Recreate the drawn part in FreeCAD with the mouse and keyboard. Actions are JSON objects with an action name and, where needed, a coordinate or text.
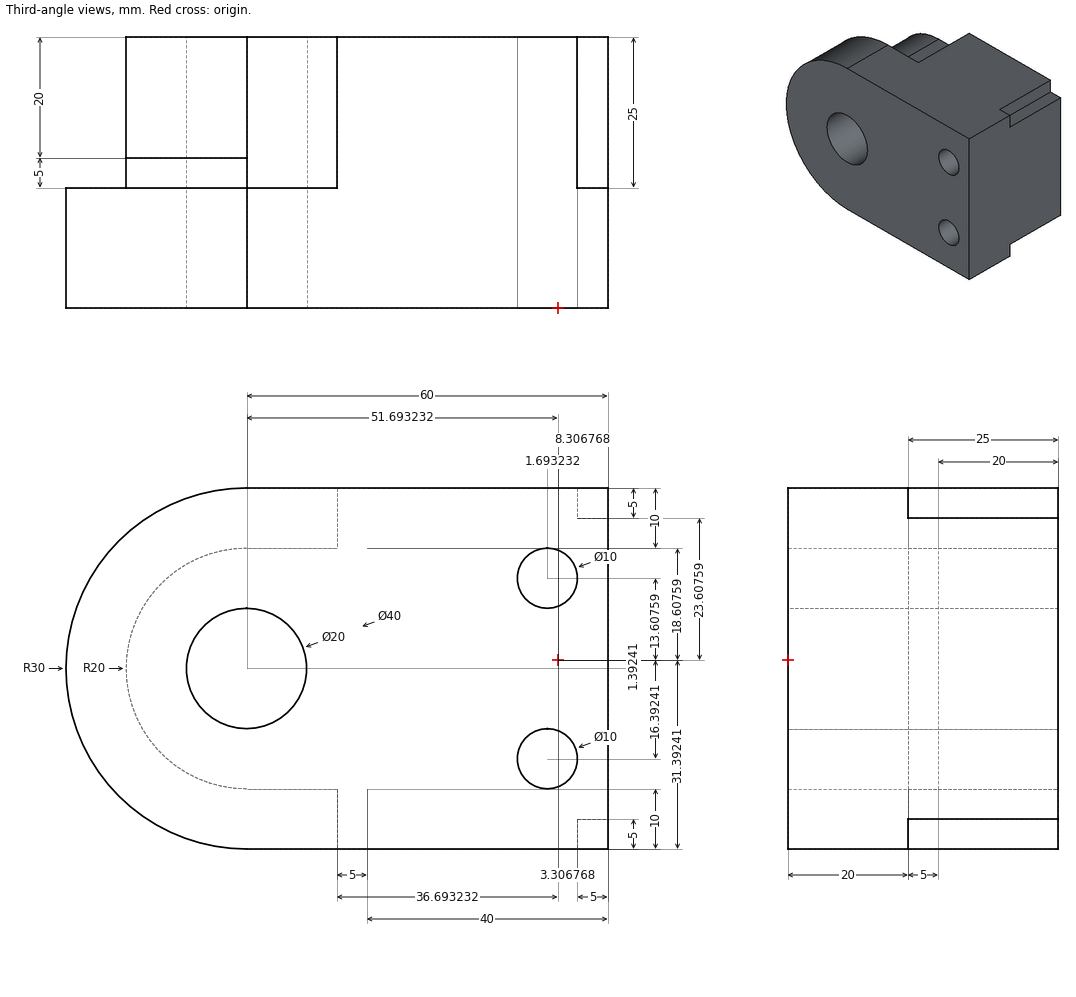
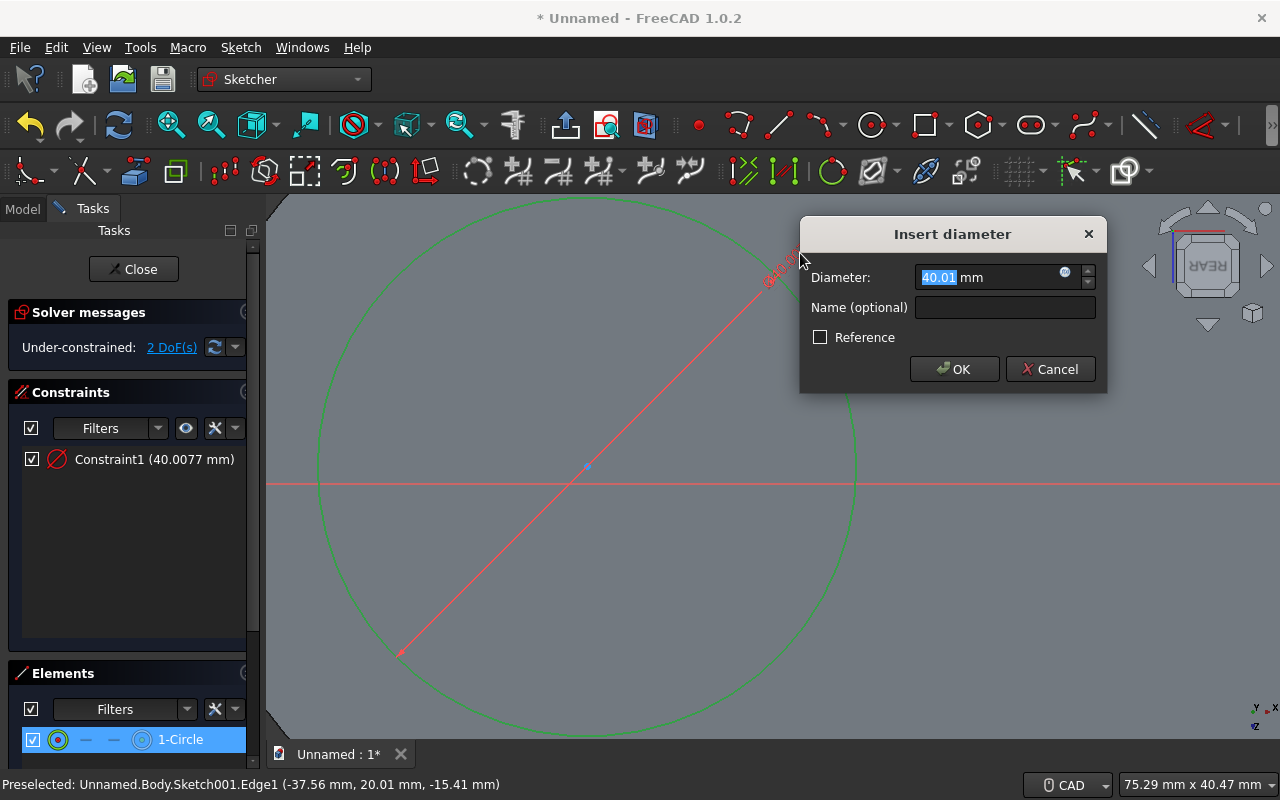
{"action": "type", "text": "40"}
{"action": "key", "text": "Return"}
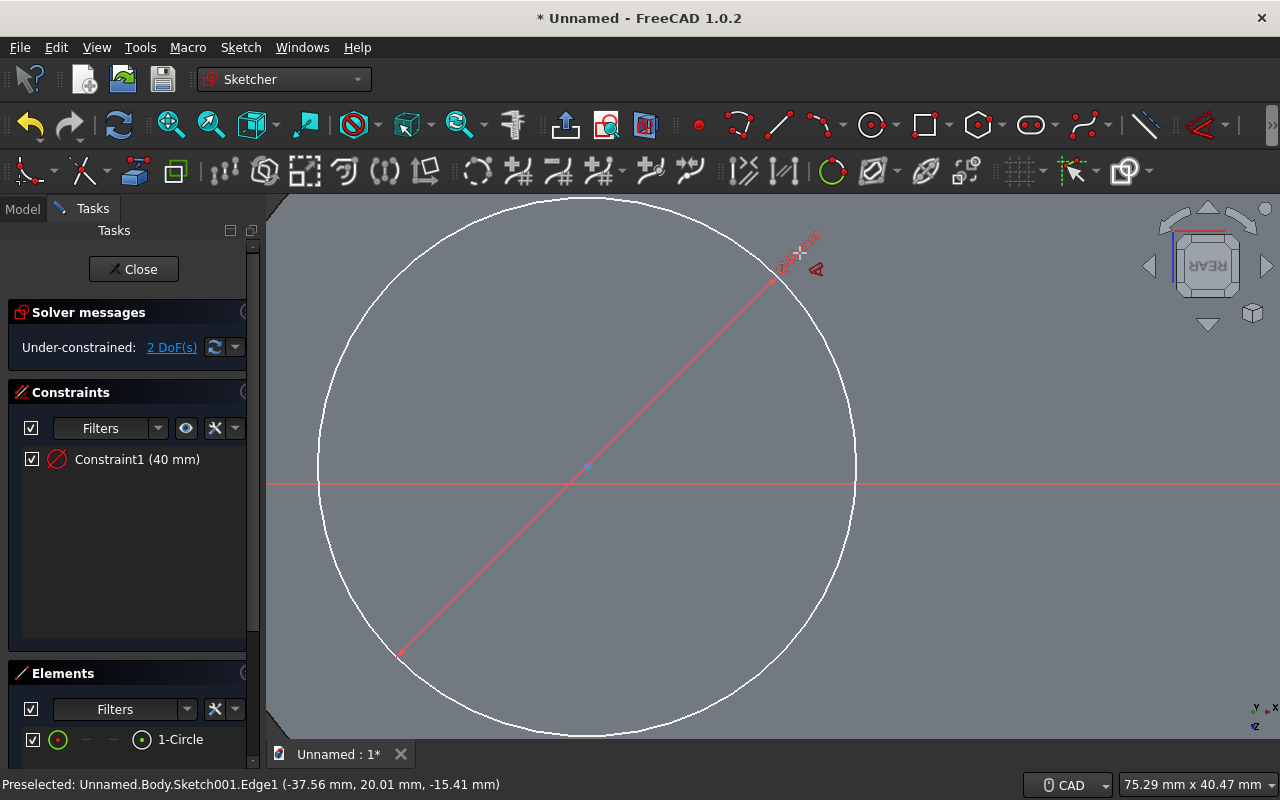
{"action": "scroll", "coordinate": [587, 467], "scroll_direction": "up", "scroll_amount": 4}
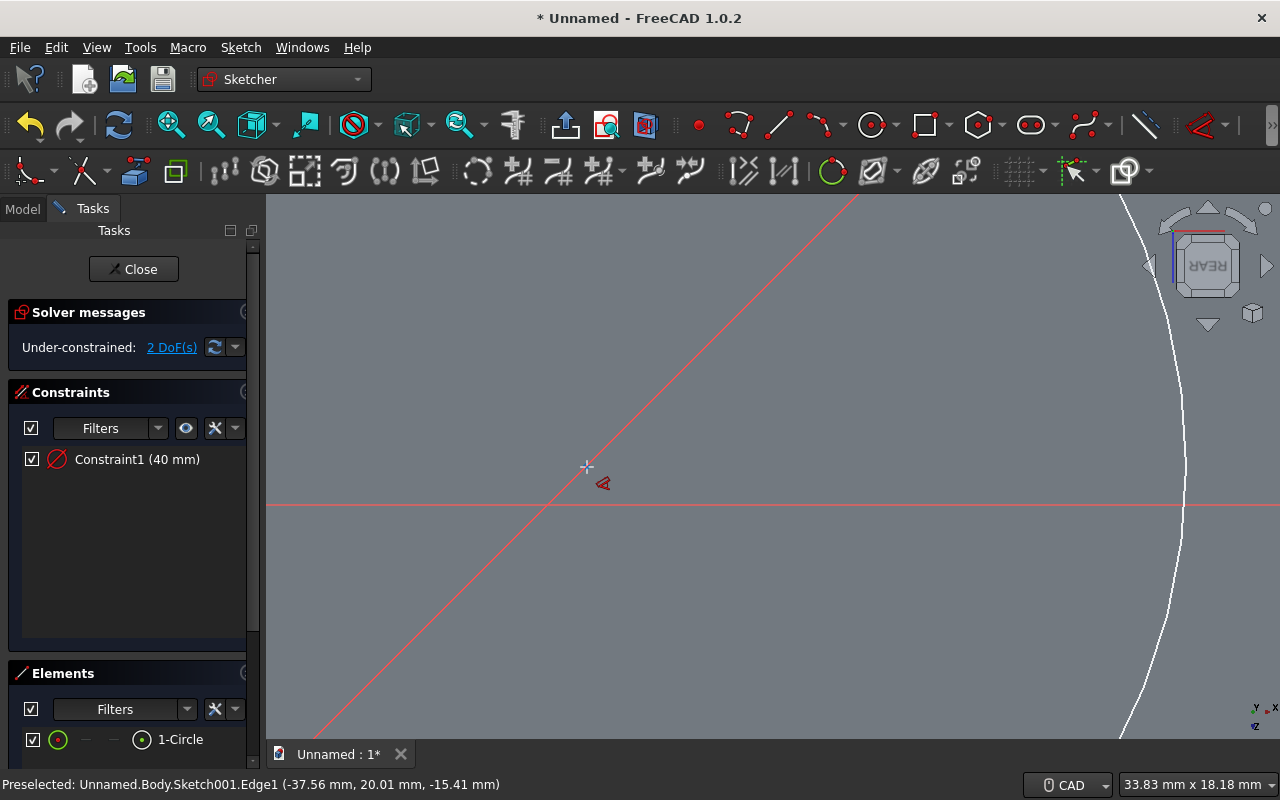
{"action": "left_click", "coordinate": [587, 466]}
{"action": "left_click", "coordinate": [553, 486]}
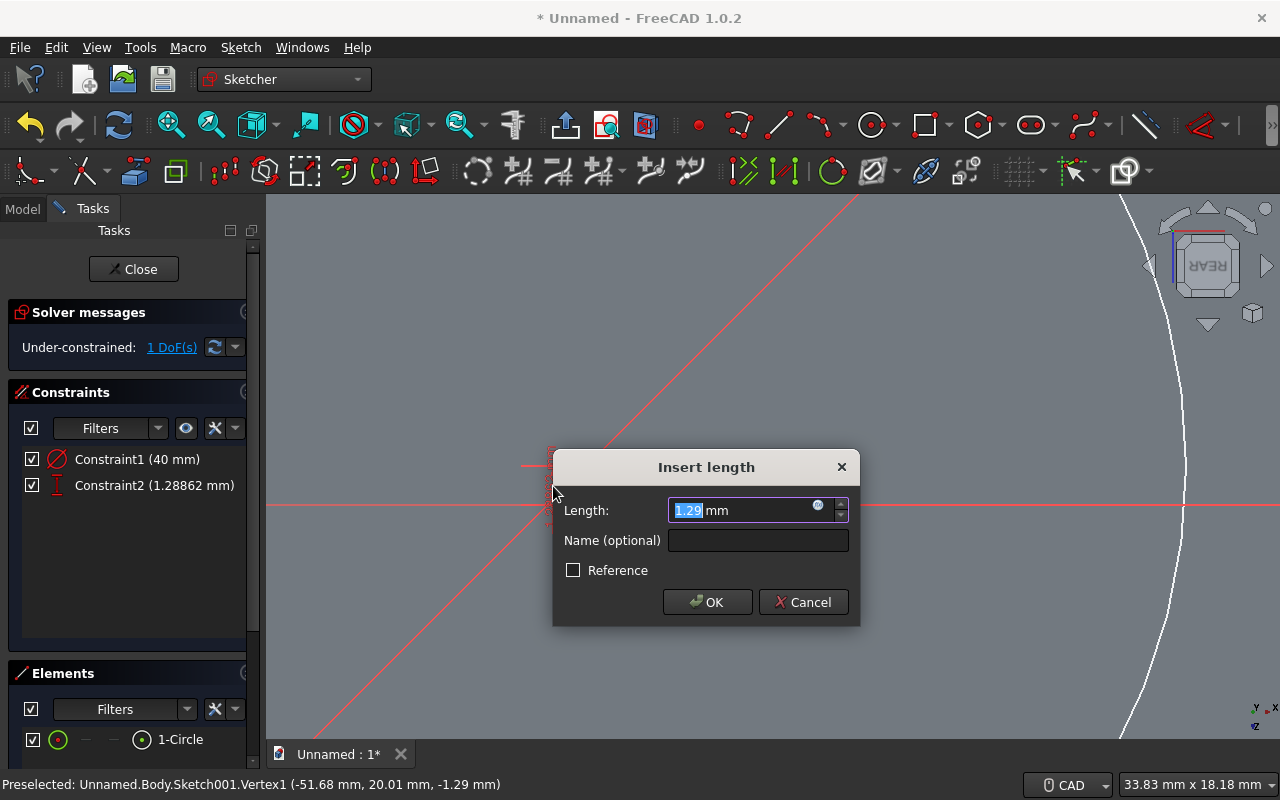
{"action": "type", "text": "1.39241"}
{"action": "key", "text": "Return"}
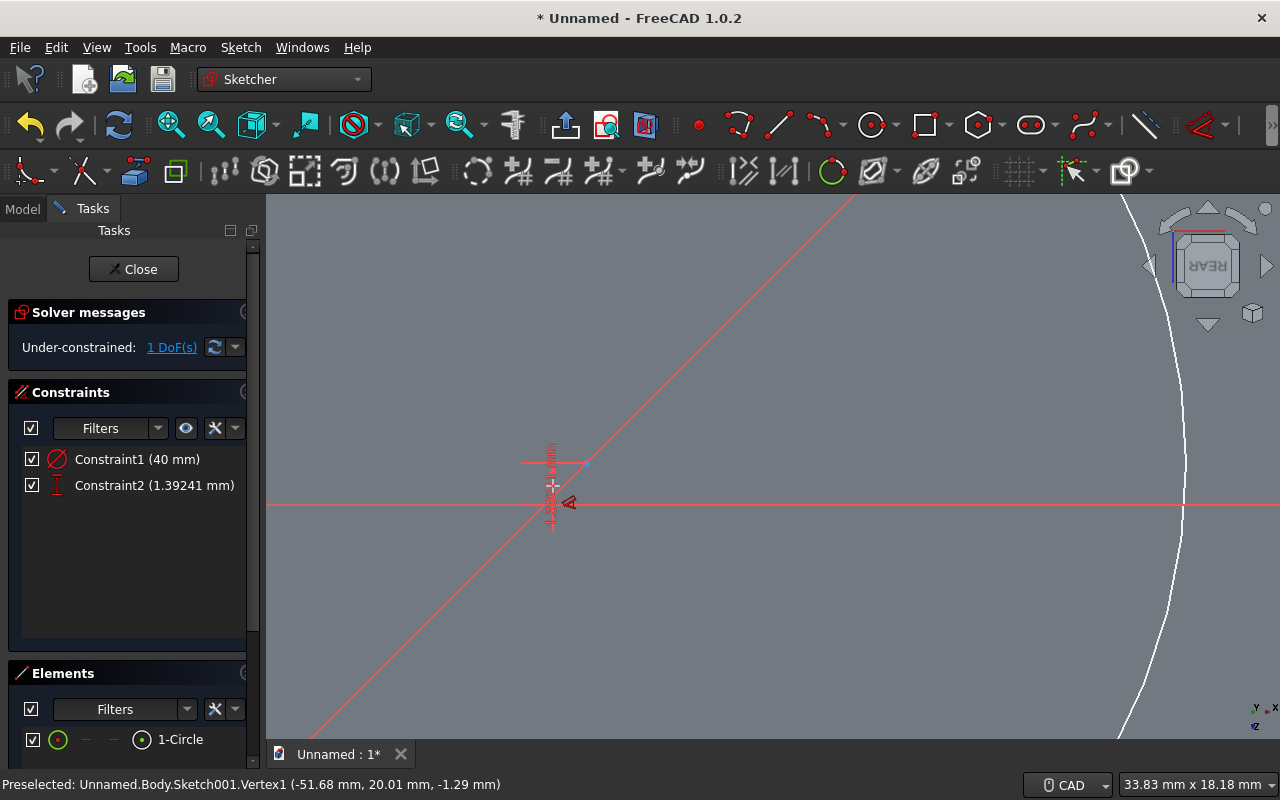
{"action": "scroll", "coordinate": [588, 468], "scroll_direction": "down", "scroll_amount": 7}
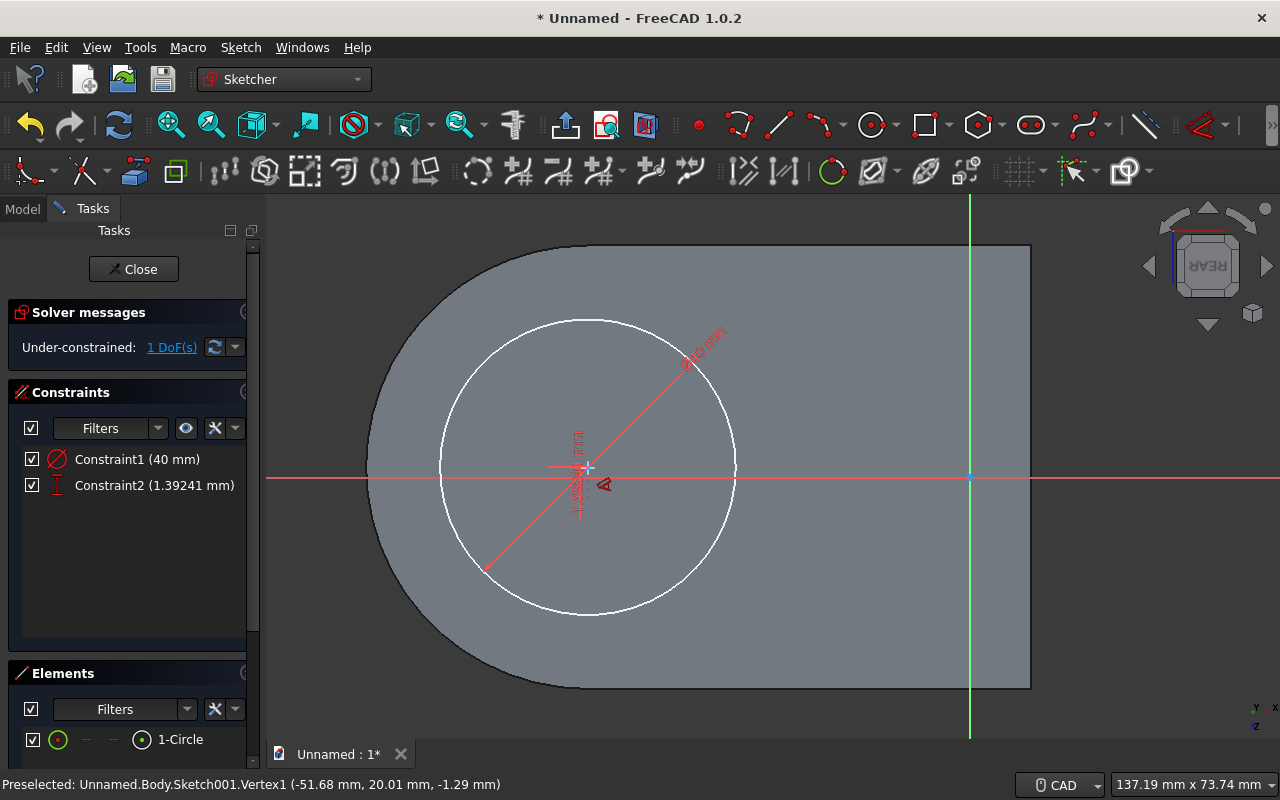
{"action": "left_click", "coordinate": [588, 467]}
{"action": "left_click", "coordinate": [779, 512]}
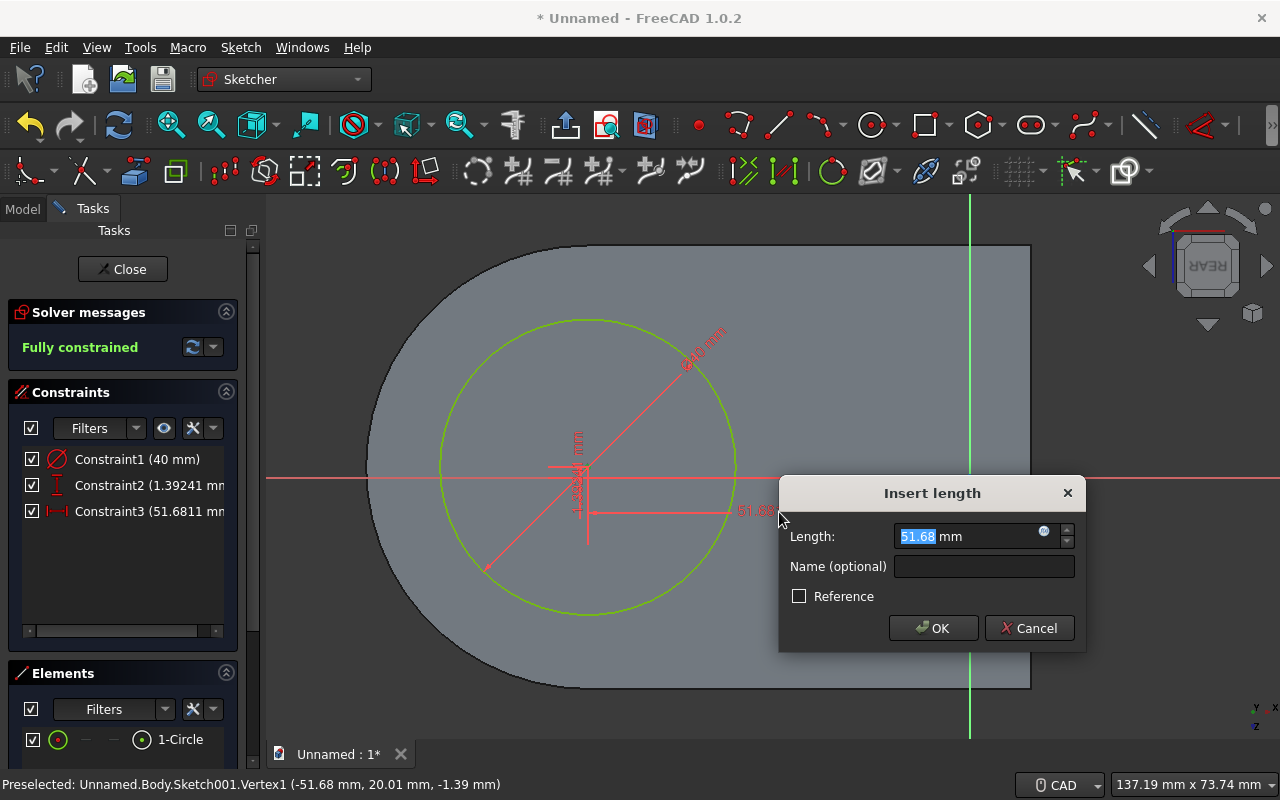
{"action": "type", "text": "51.693232"}
{"action": "key", "text": "Return"}
{"action": "key", "text": "Escape"}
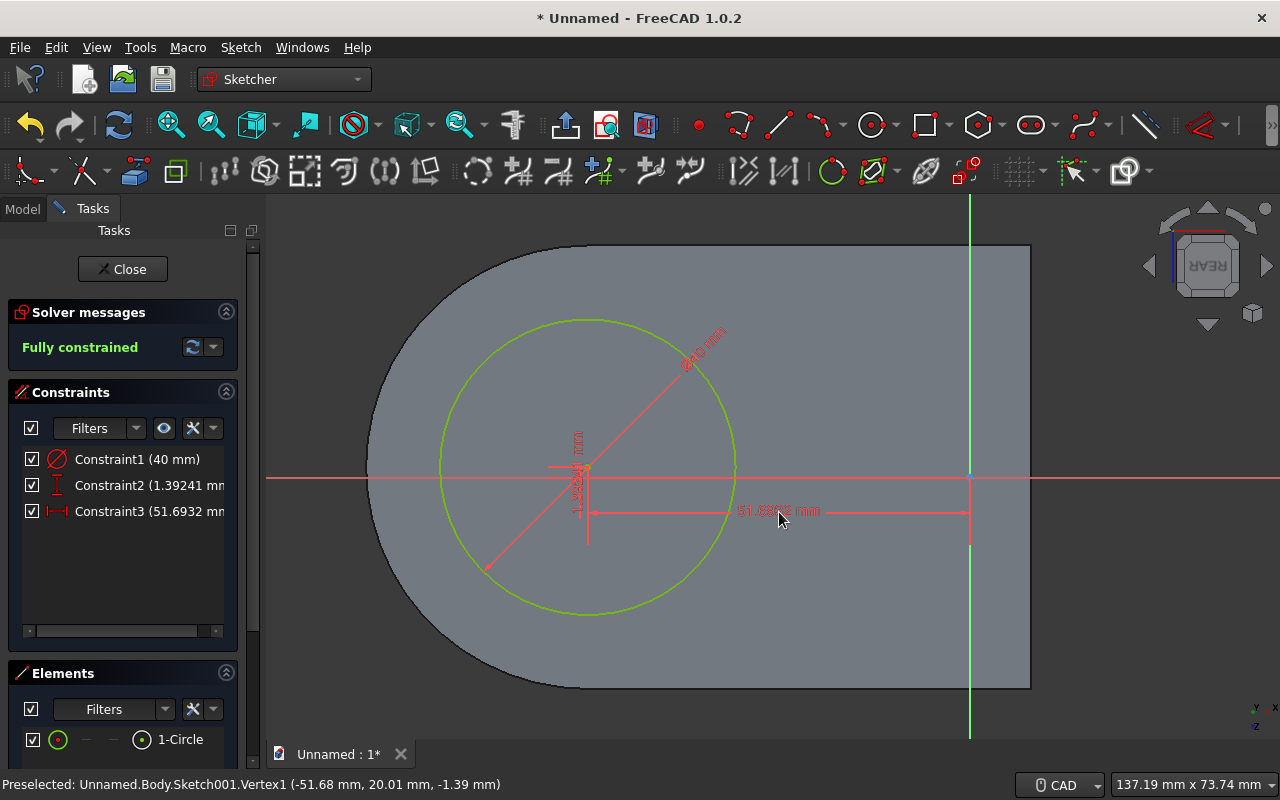
{"action": "left_click", "coordinate": [123, 269]}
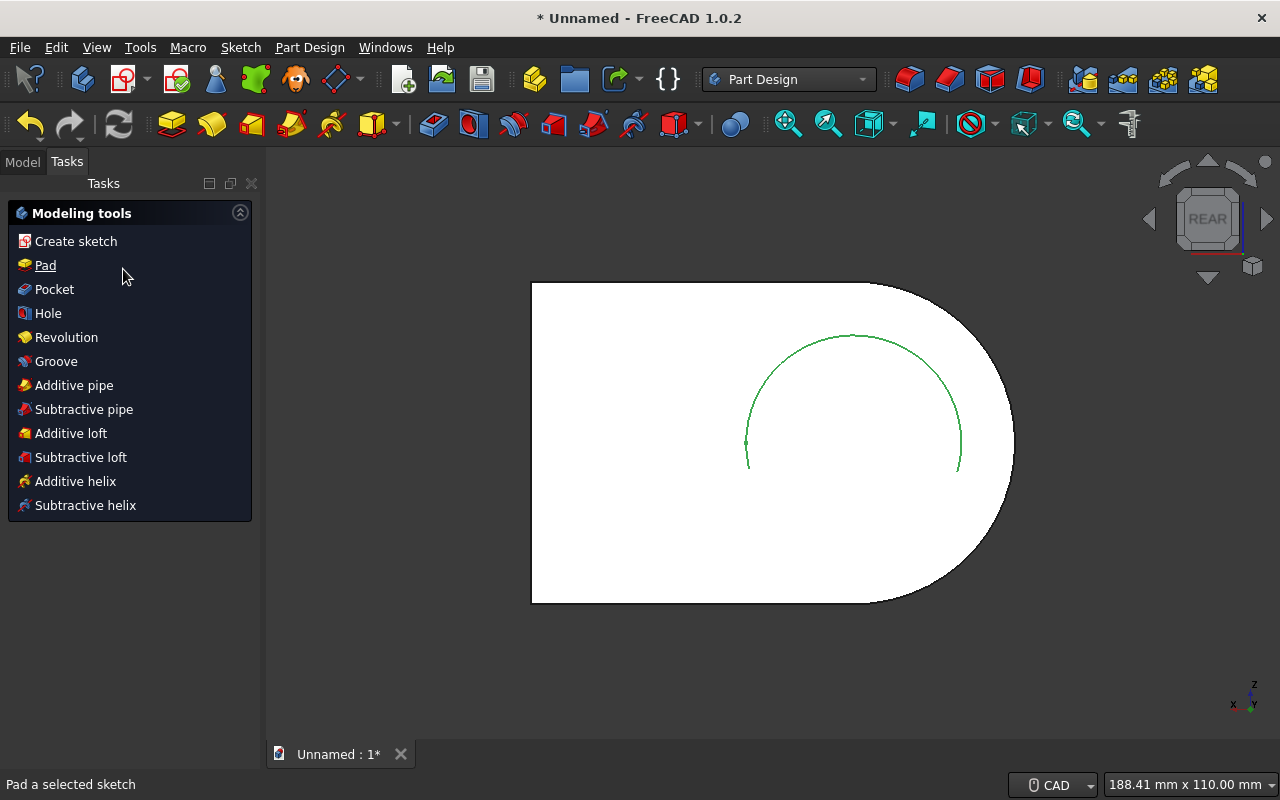
{"action": "left_click", "coordinate": [172, 124]}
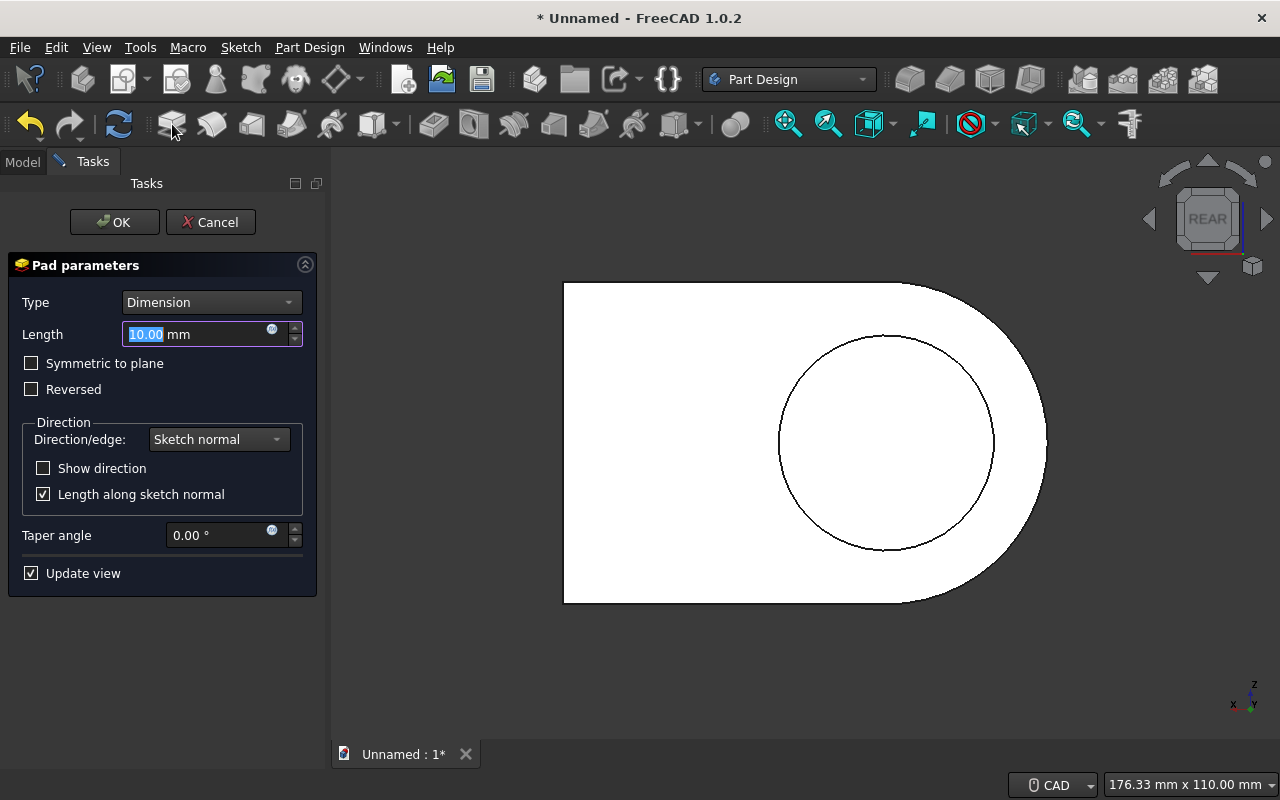
{"action": "type", "text": "5"}
{"action": "key", "text": "Tab"}